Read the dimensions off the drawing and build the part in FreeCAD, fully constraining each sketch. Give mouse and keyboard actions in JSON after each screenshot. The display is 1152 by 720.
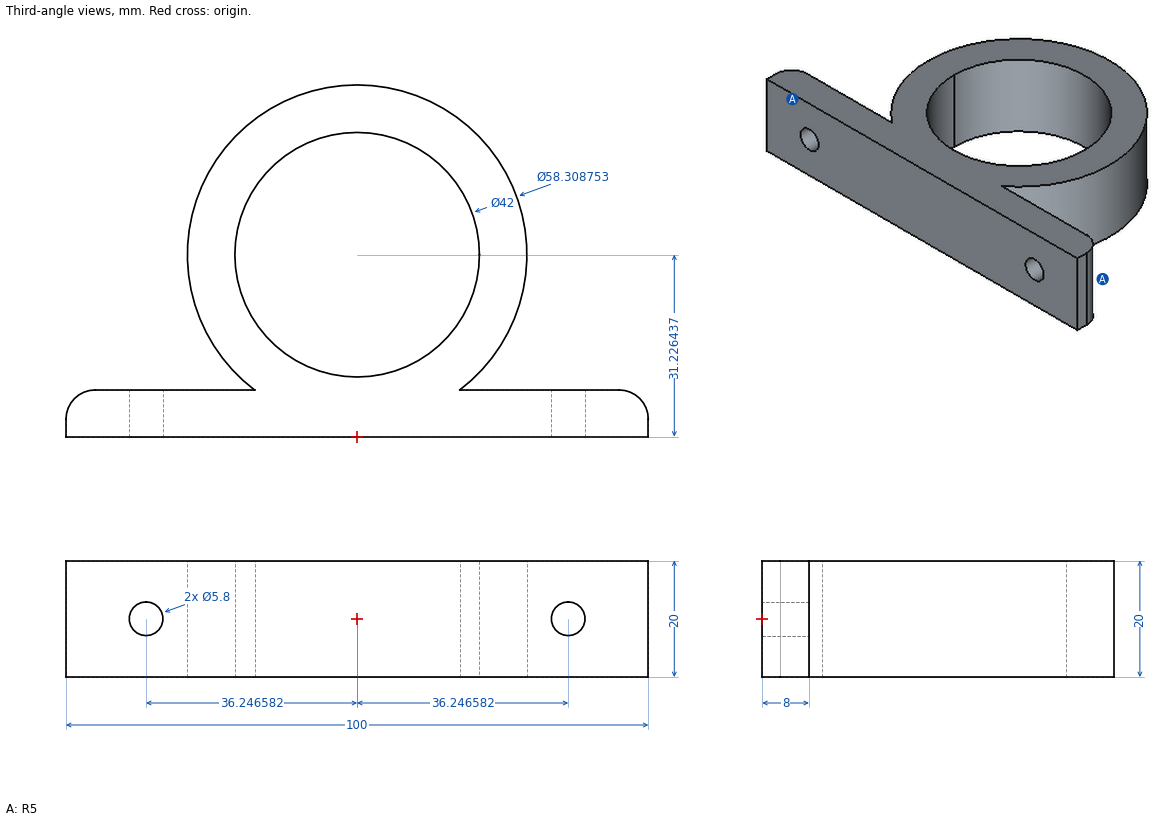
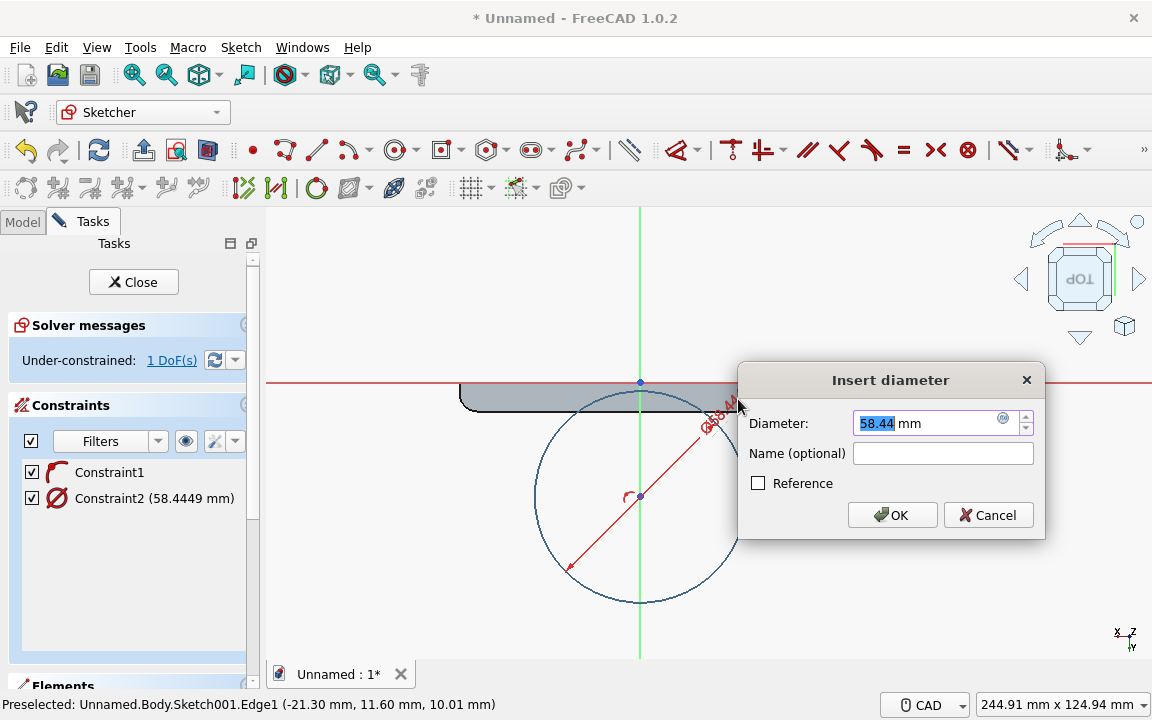
{"action": "type", "text": "58.308753"}
{"action": "key", "text": "Return"}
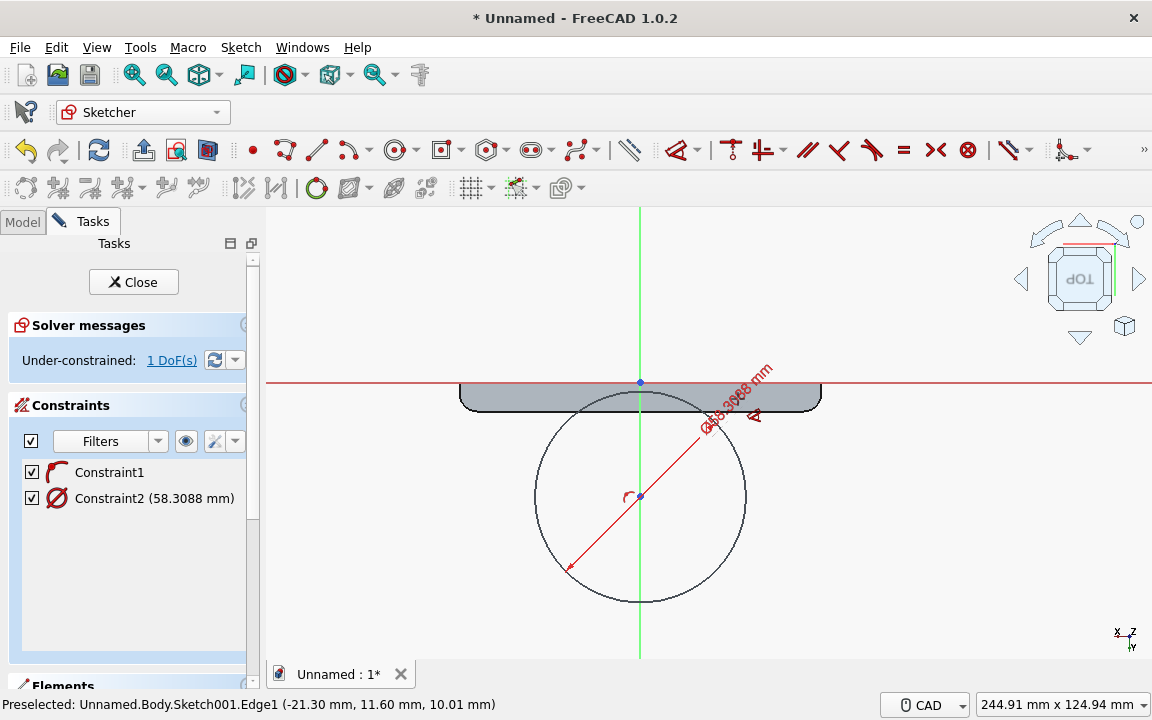
{"action": "left_click", "coordinate": [640, 497]}
{"action": "left_click", "coordinate": [674, 440]}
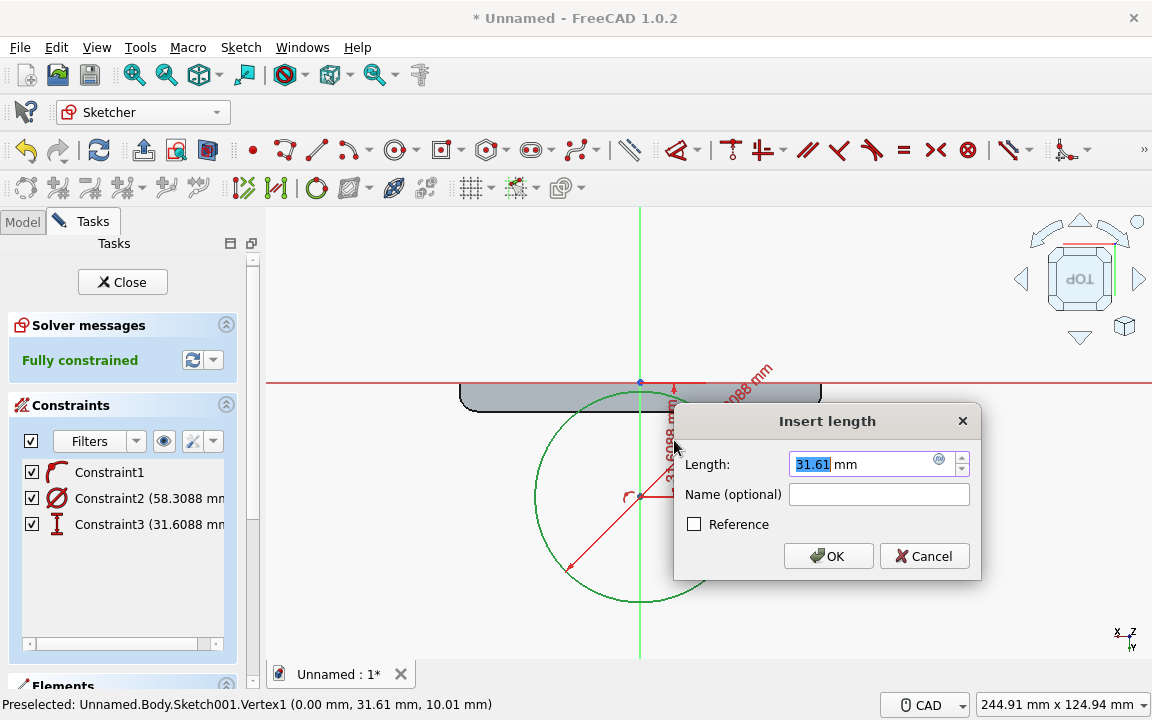
{"action": "type", "text": "31.226437"}
{"action": "key", "text": "Return"}
{"action": "key", "text": "Escape"}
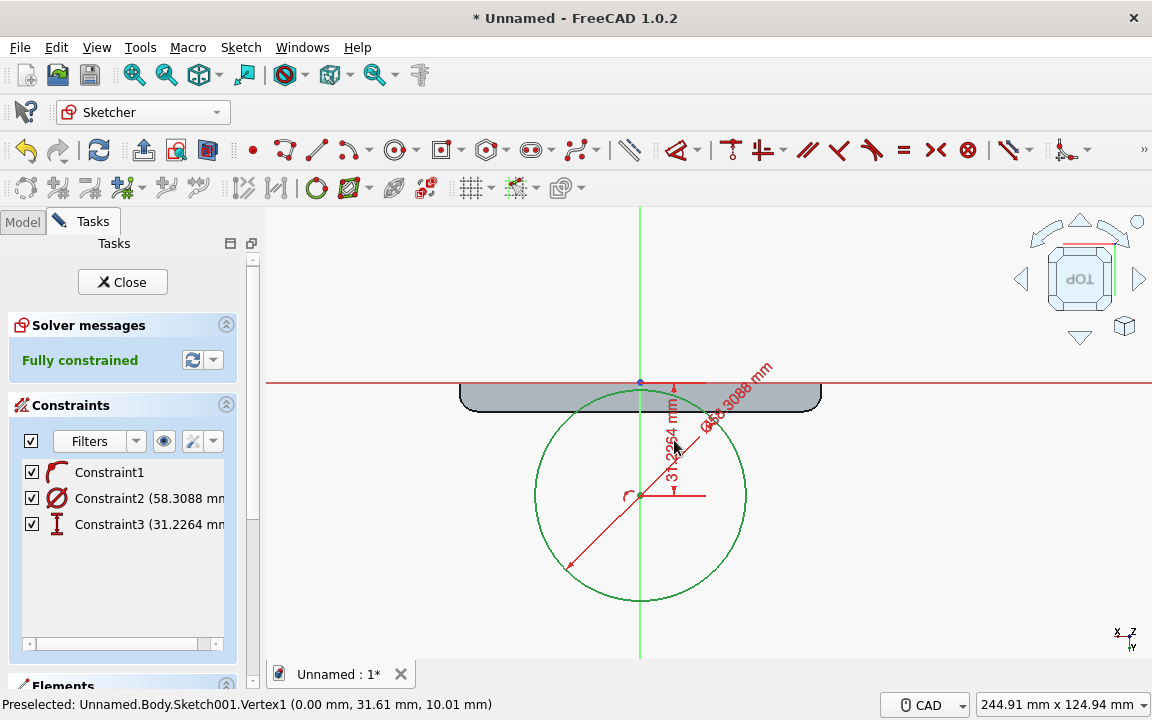
{"action": "left_click", "coordinate": [123, 282]}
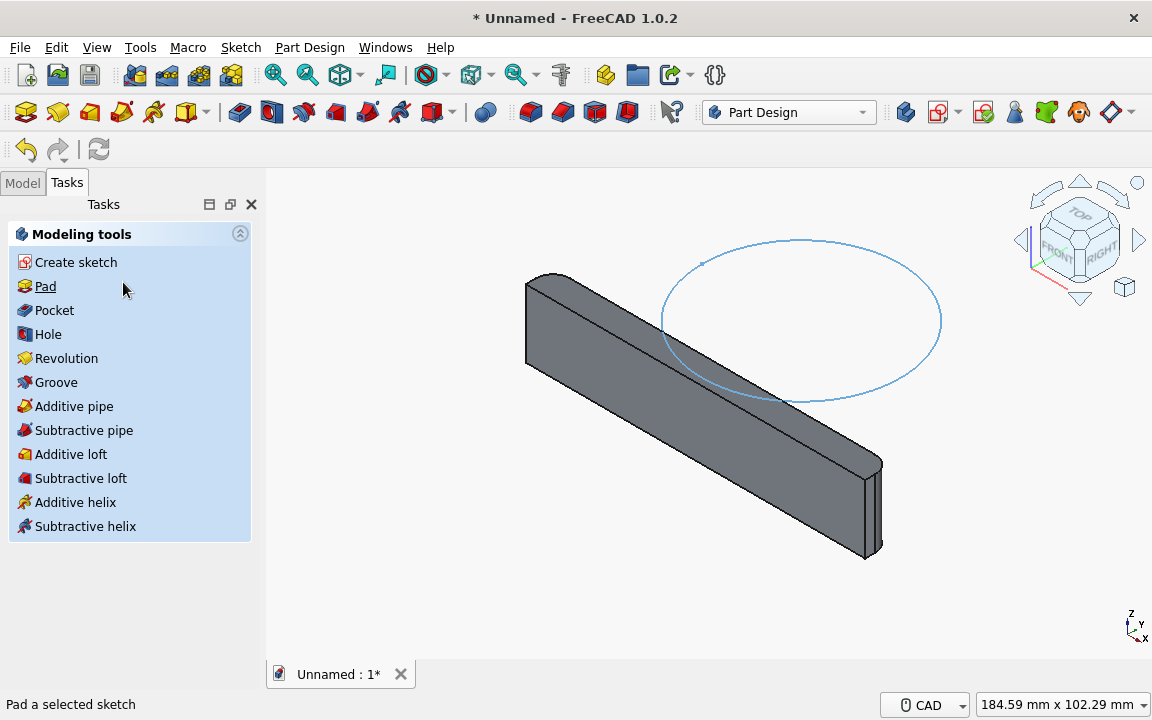
{"action": "left_click", "coordinate": [26, 112]}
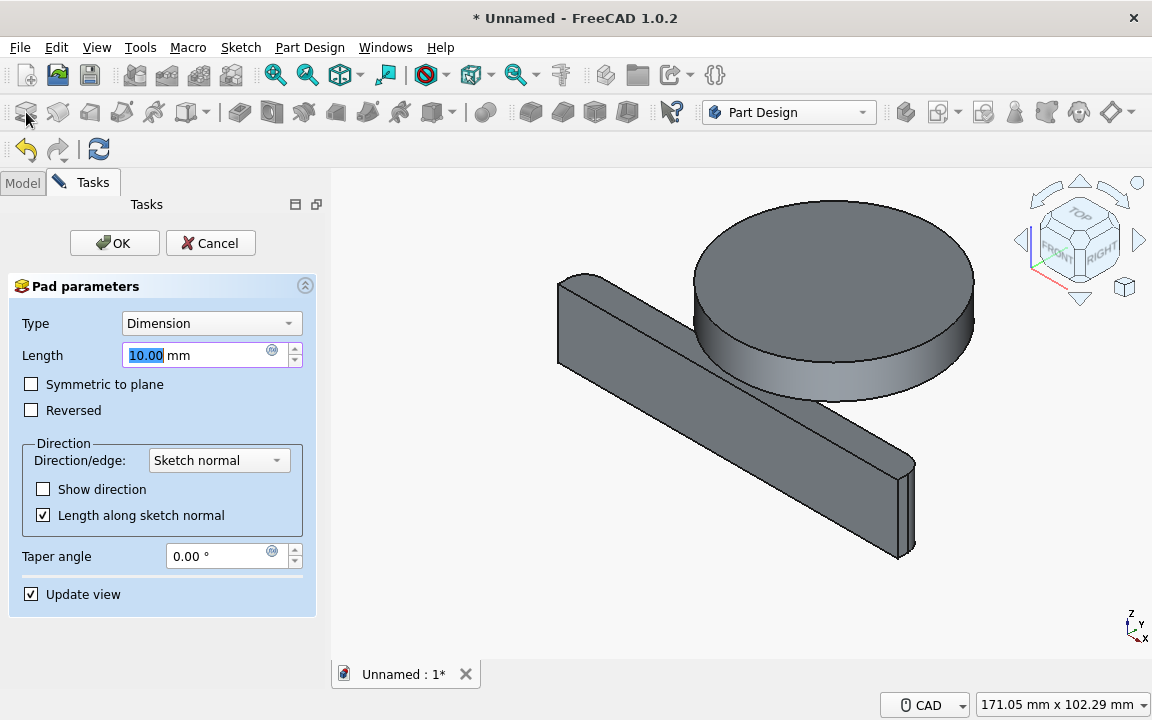
{"action": "type", "text": "20"}
{"action": "key", "text": "Tab"}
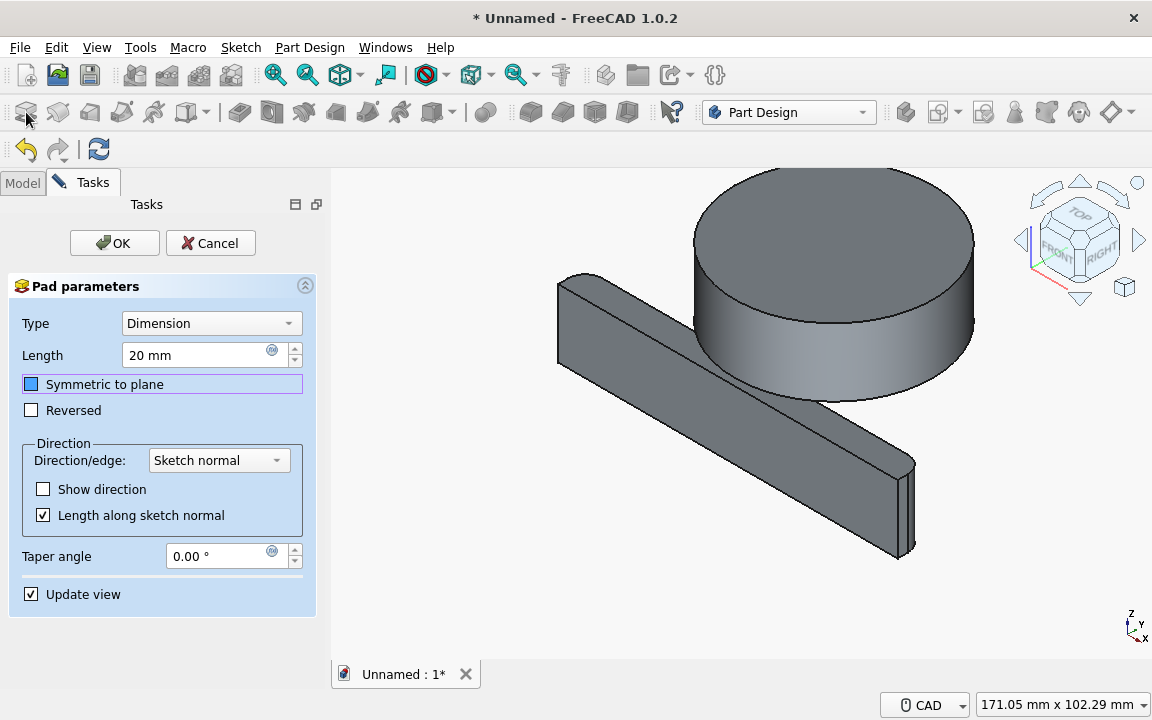
{"action": "left_click", "coordinate": [30, 410]}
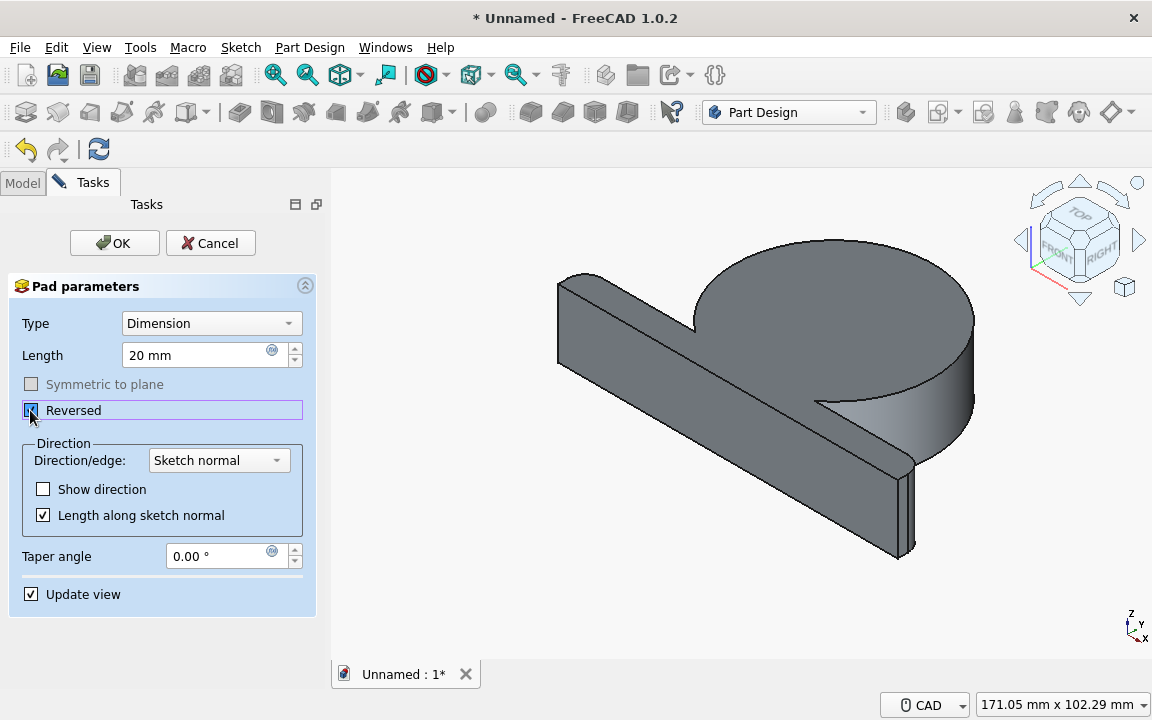
{"action": "left_click", "coordinate": [115, 243]}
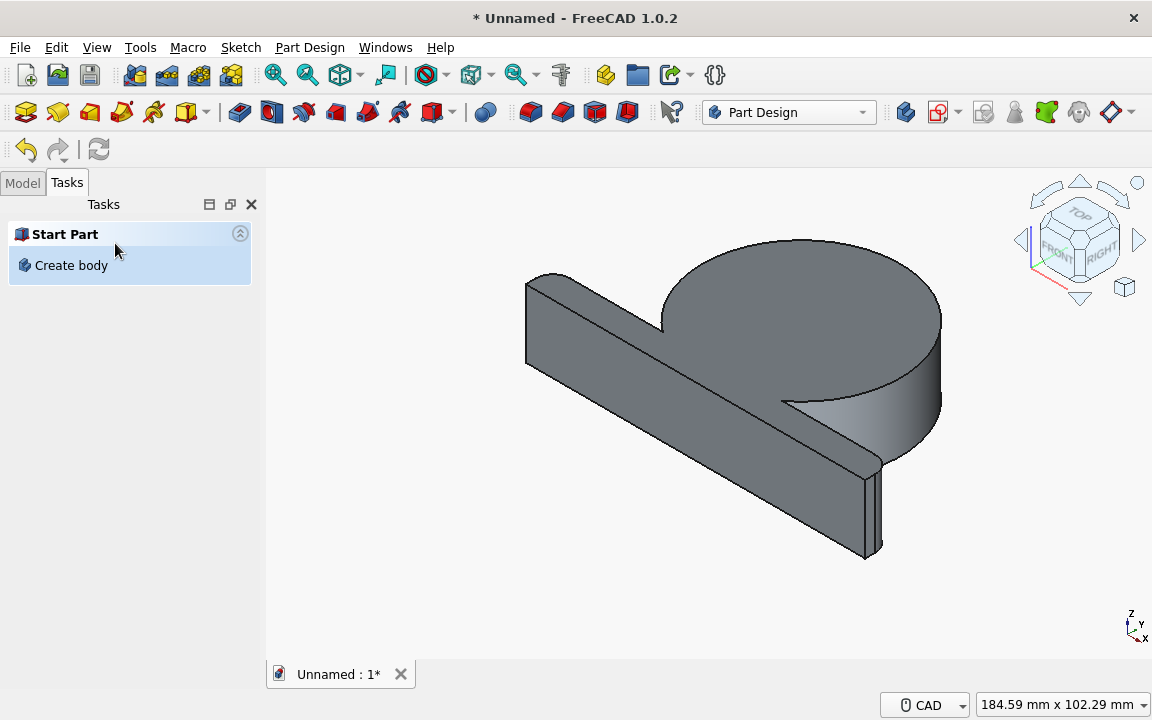
{"action": "left_click", "coordinate": [276, 76]}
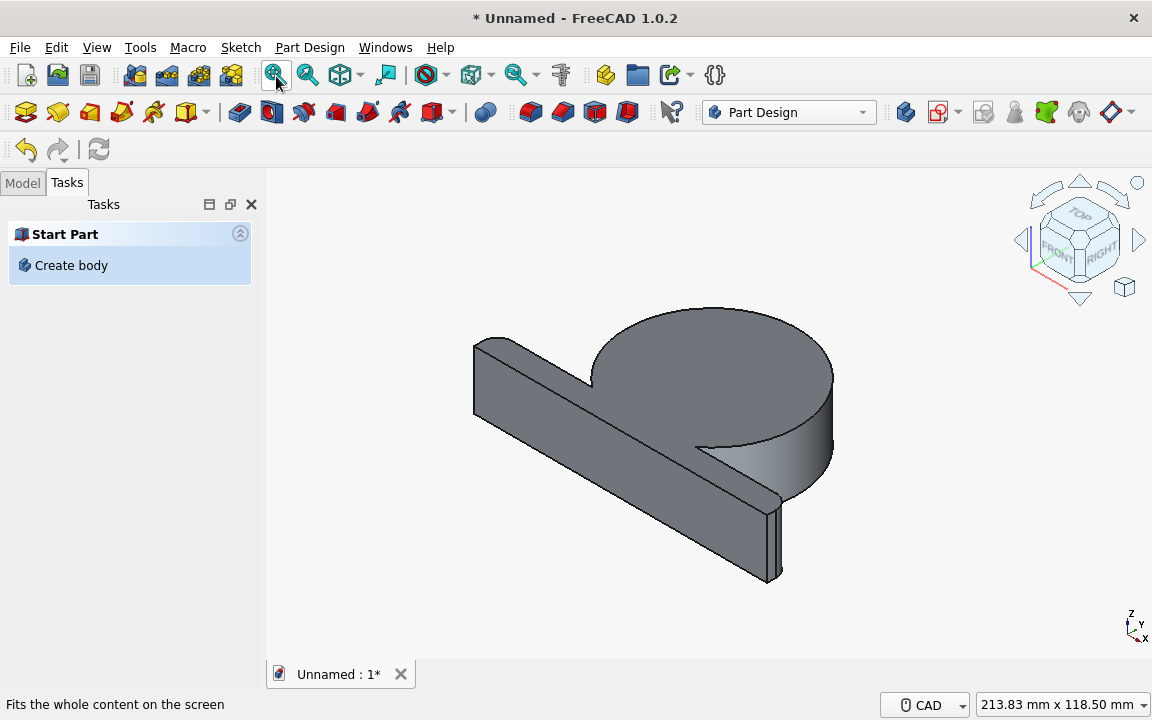
{"action": "key", "text": "4"}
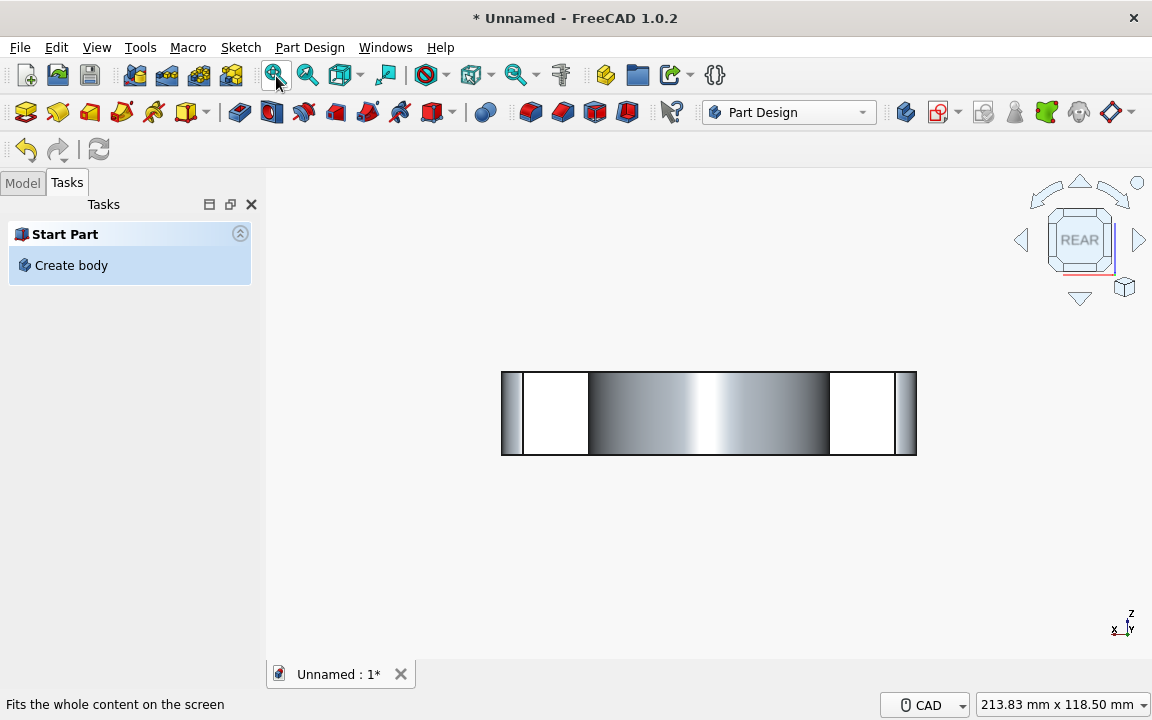
{"action": "left_click", "coordinate": [839, 413]}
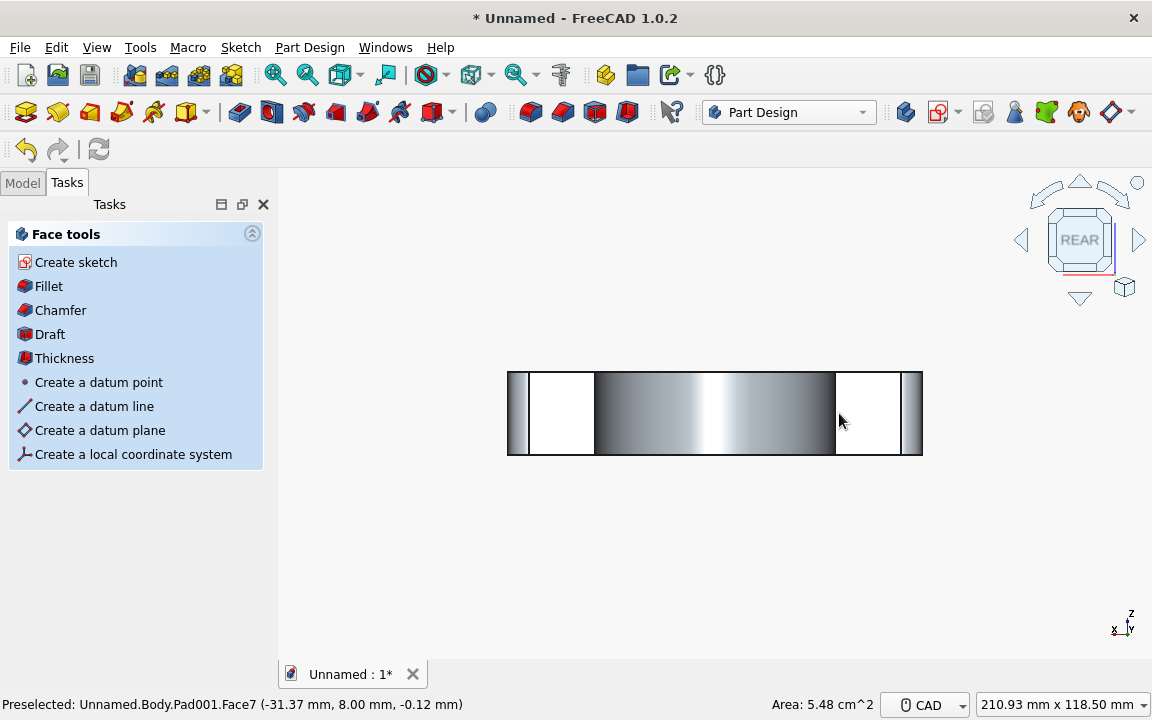
{"action": "left_click", "coordinate": [938, 112]}